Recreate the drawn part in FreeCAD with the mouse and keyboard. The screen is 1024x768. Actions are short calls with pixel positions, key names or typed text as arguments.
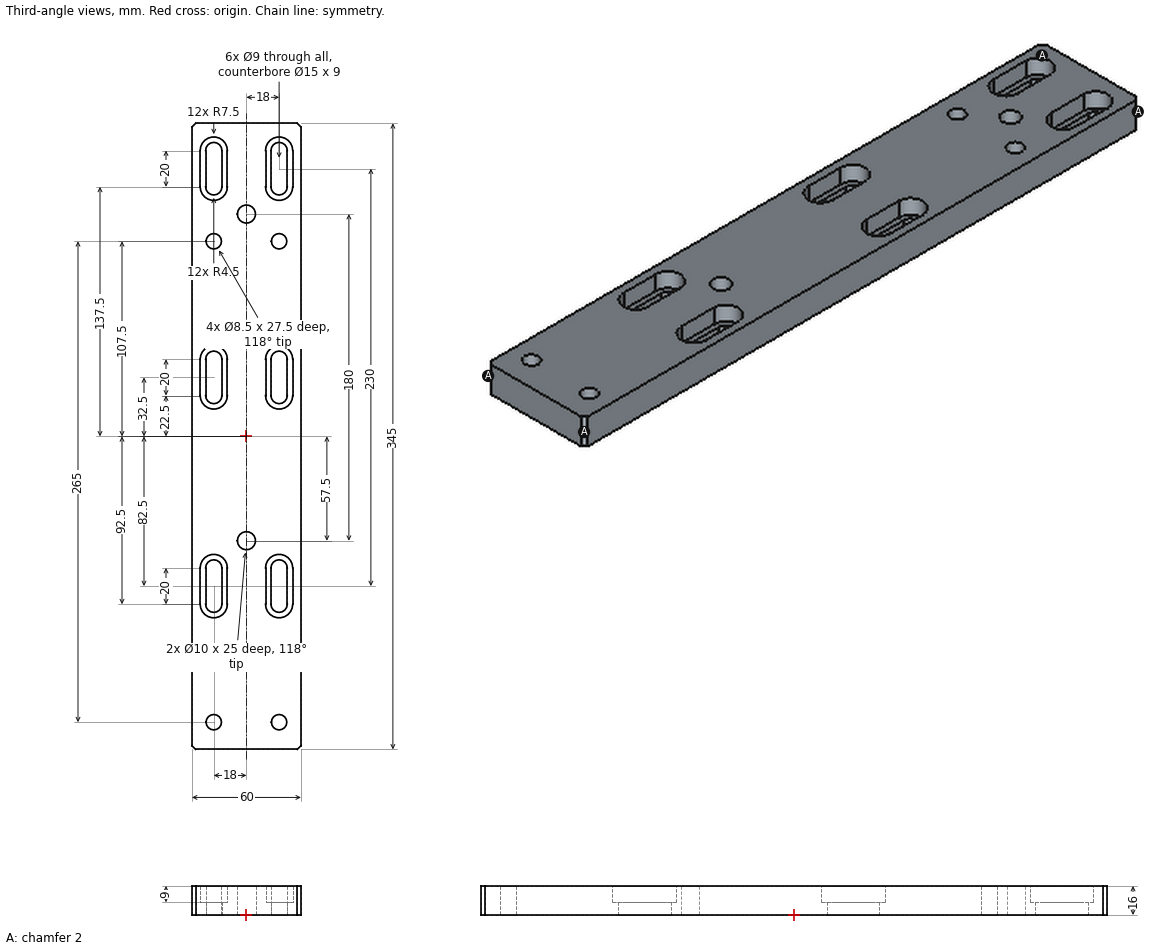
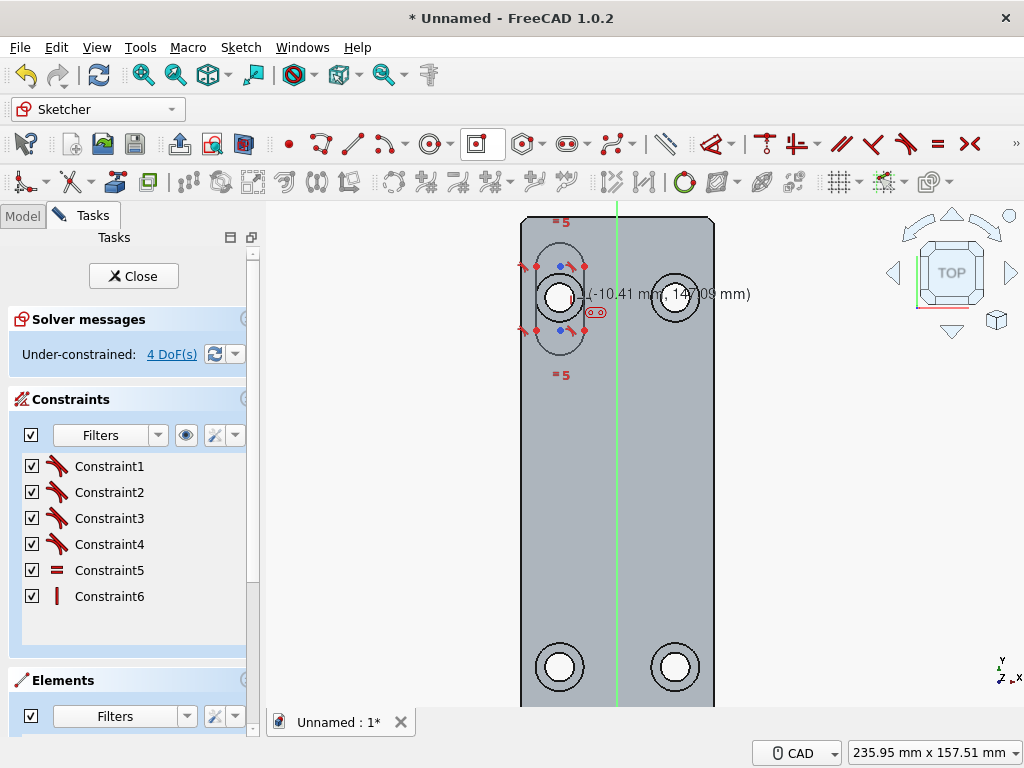
click(675, 330)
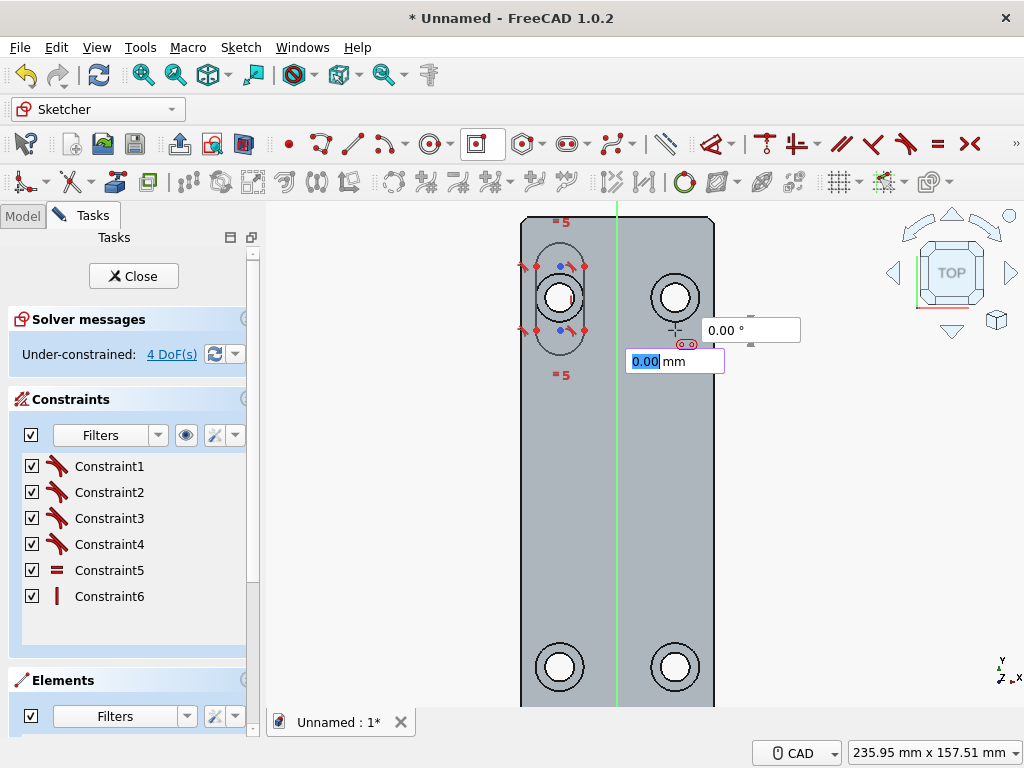
click(675, 266)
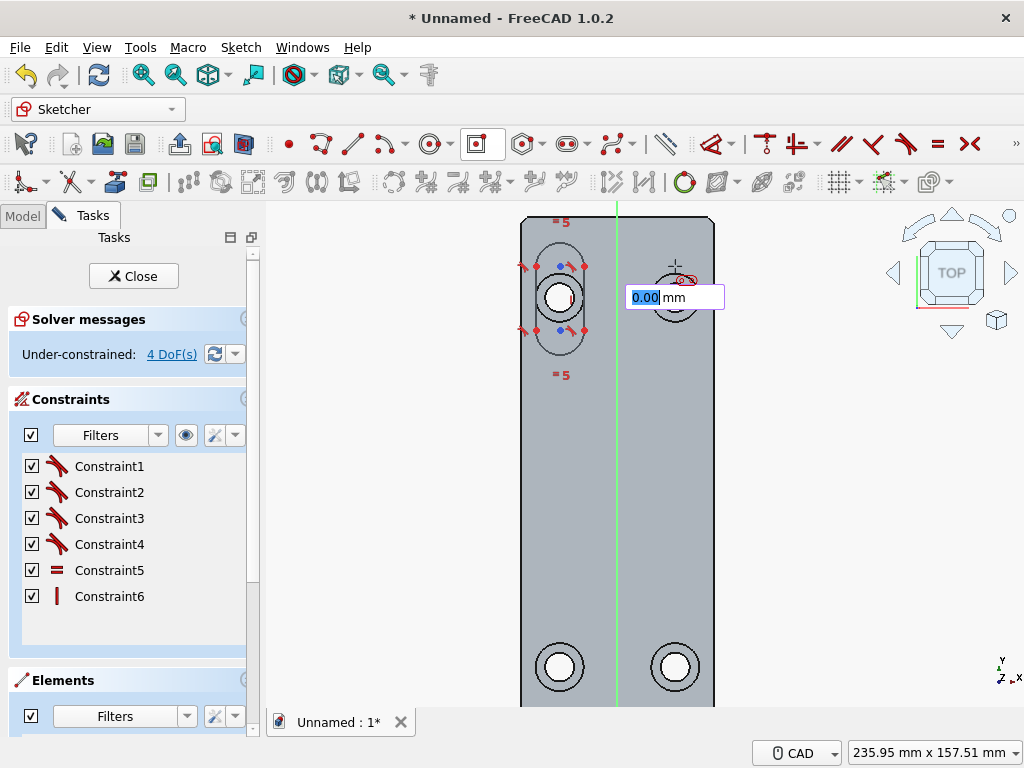
click(699, 298)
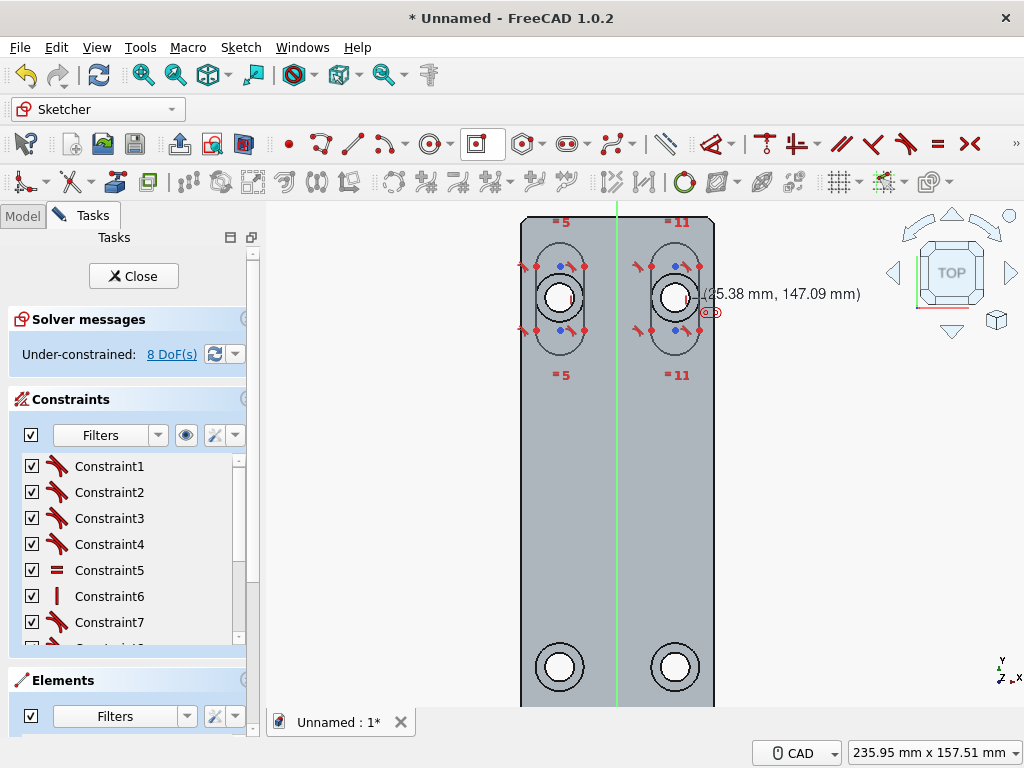
scroll(553, 330, down, 5)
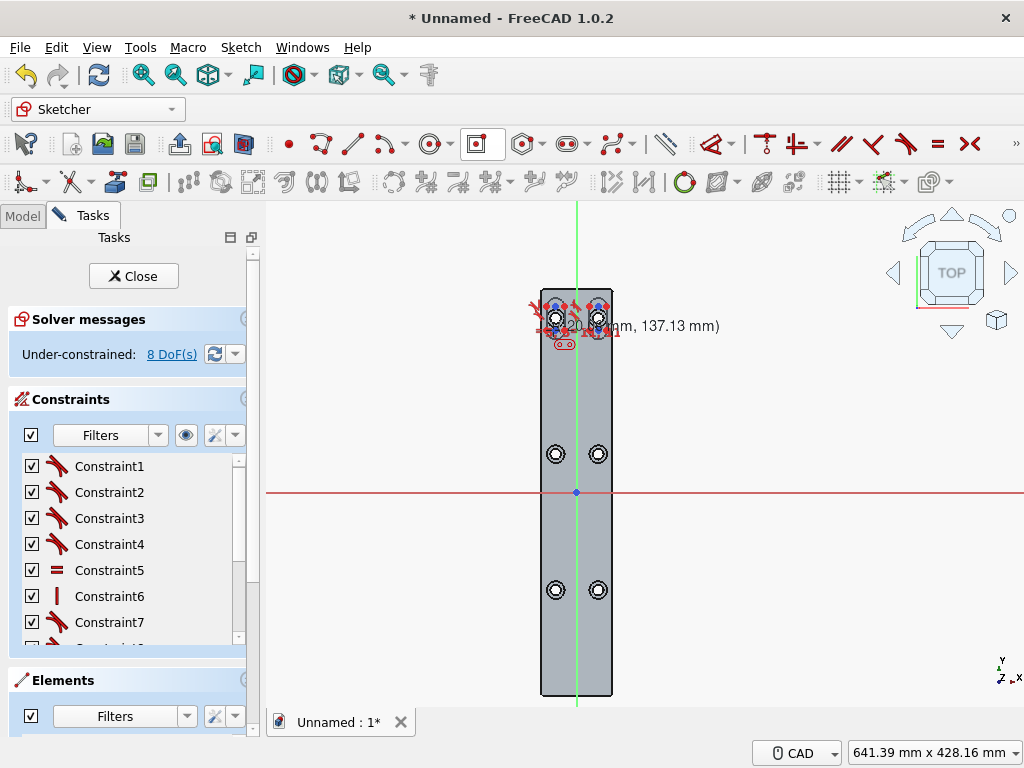
scroll(556, 466, up, 5)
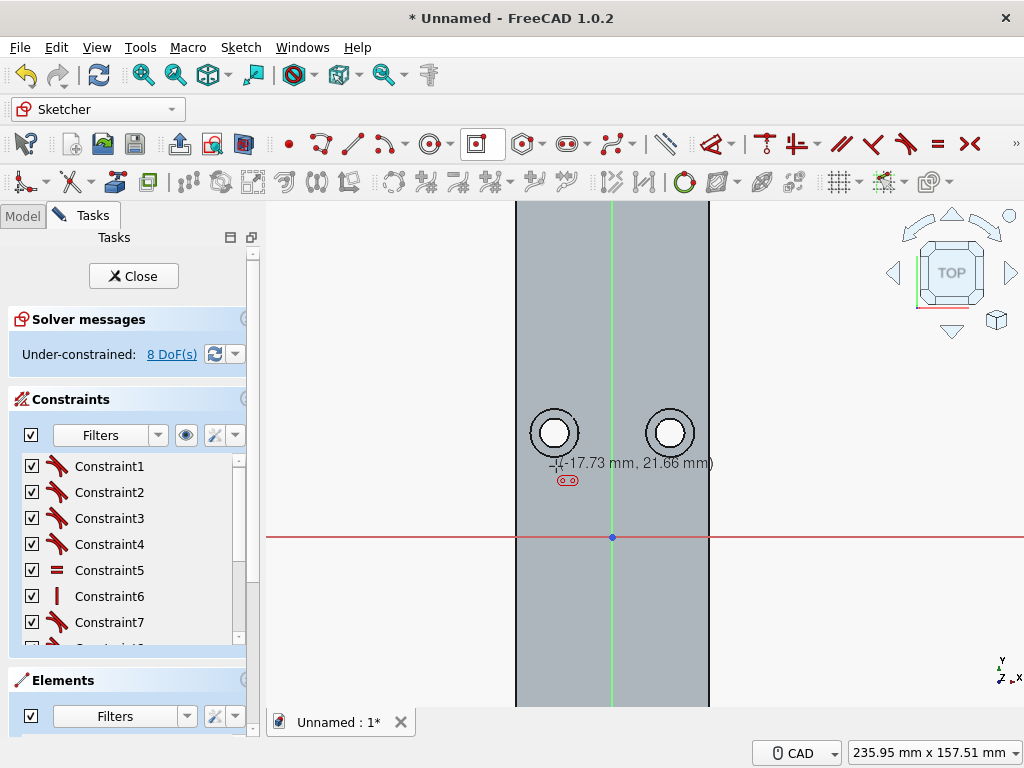
click(554, 465)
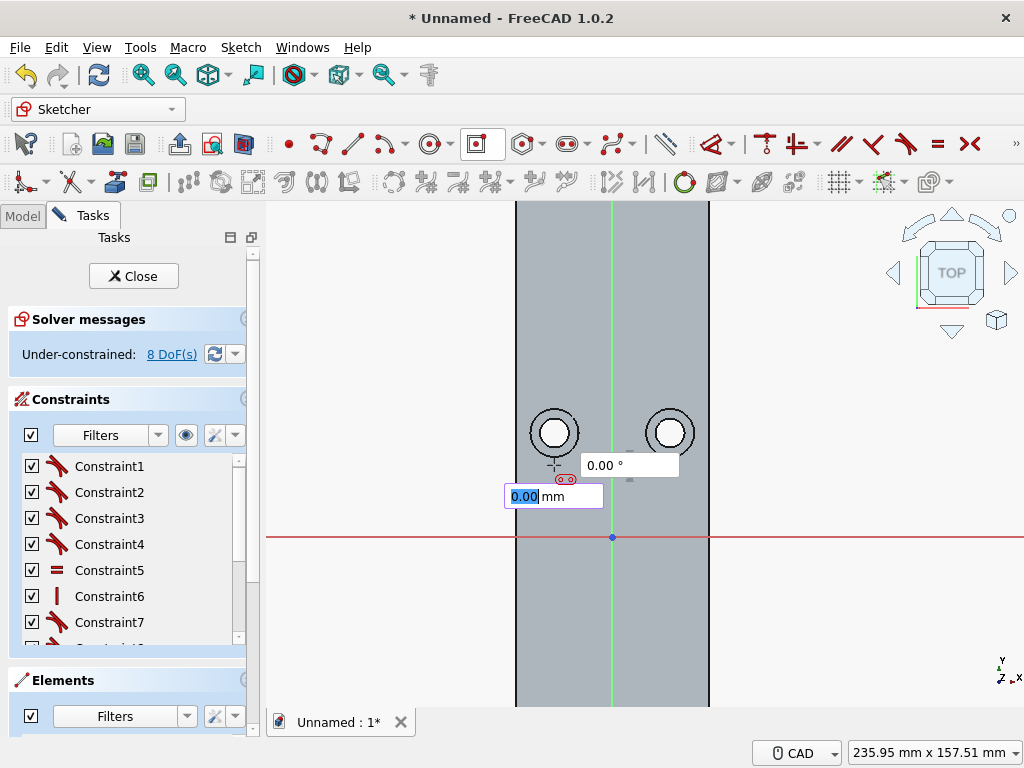
click(554, 401)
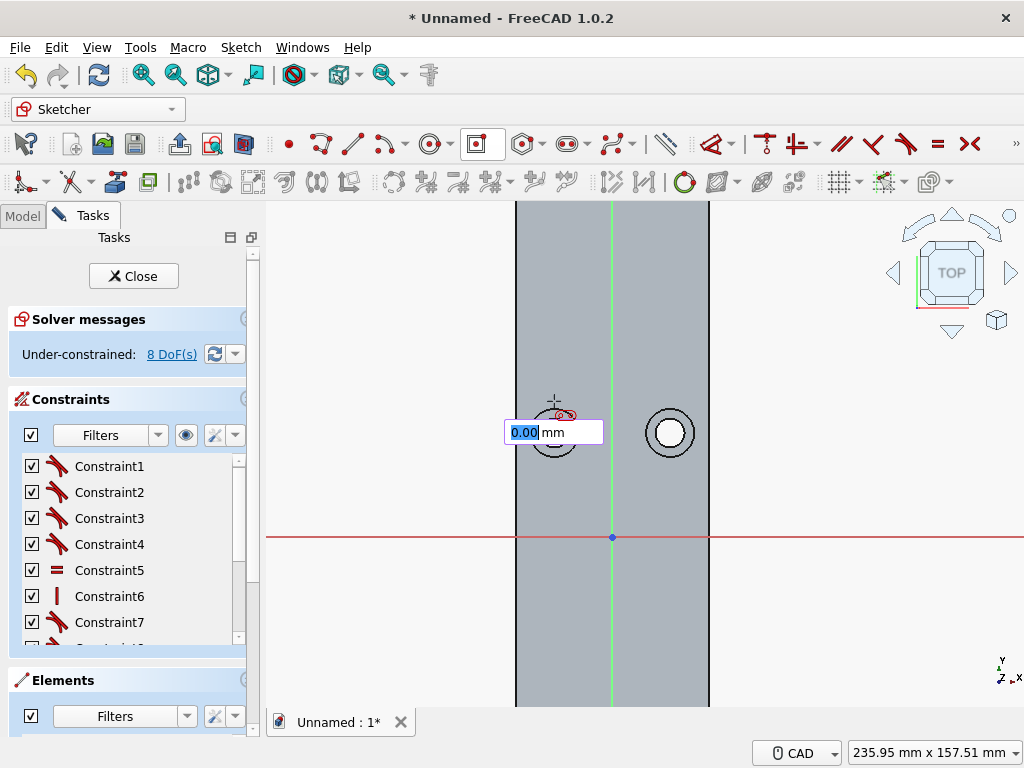
click(530, 433)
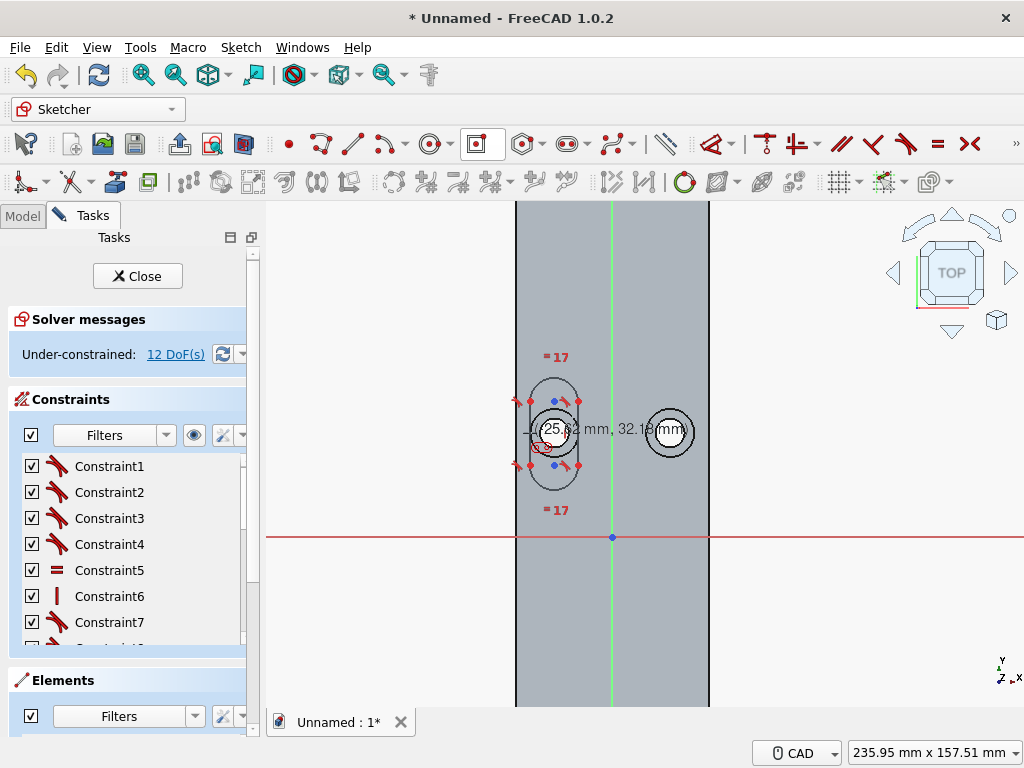
click(670, 465)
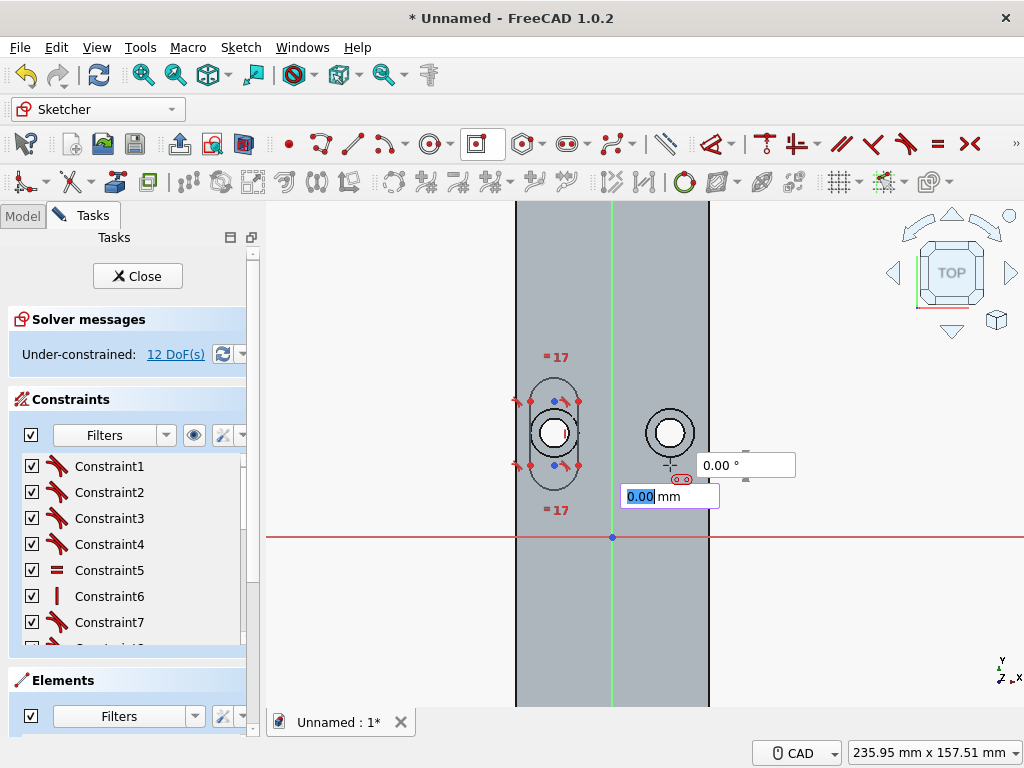
click(670, 401)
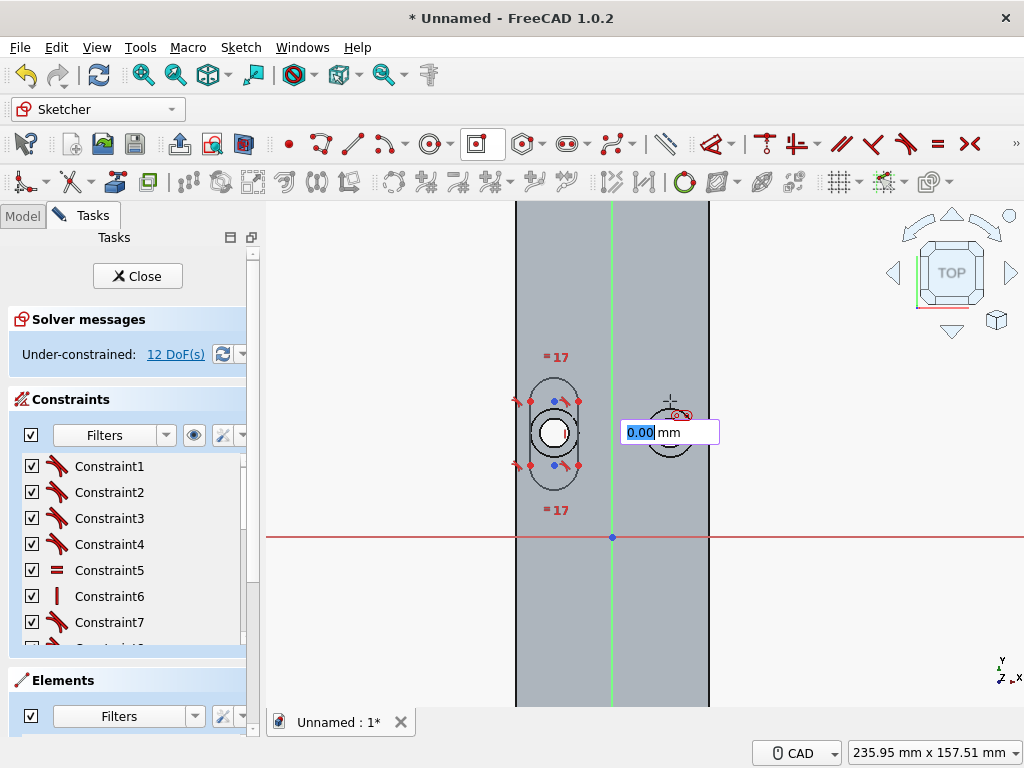
click(646, 433)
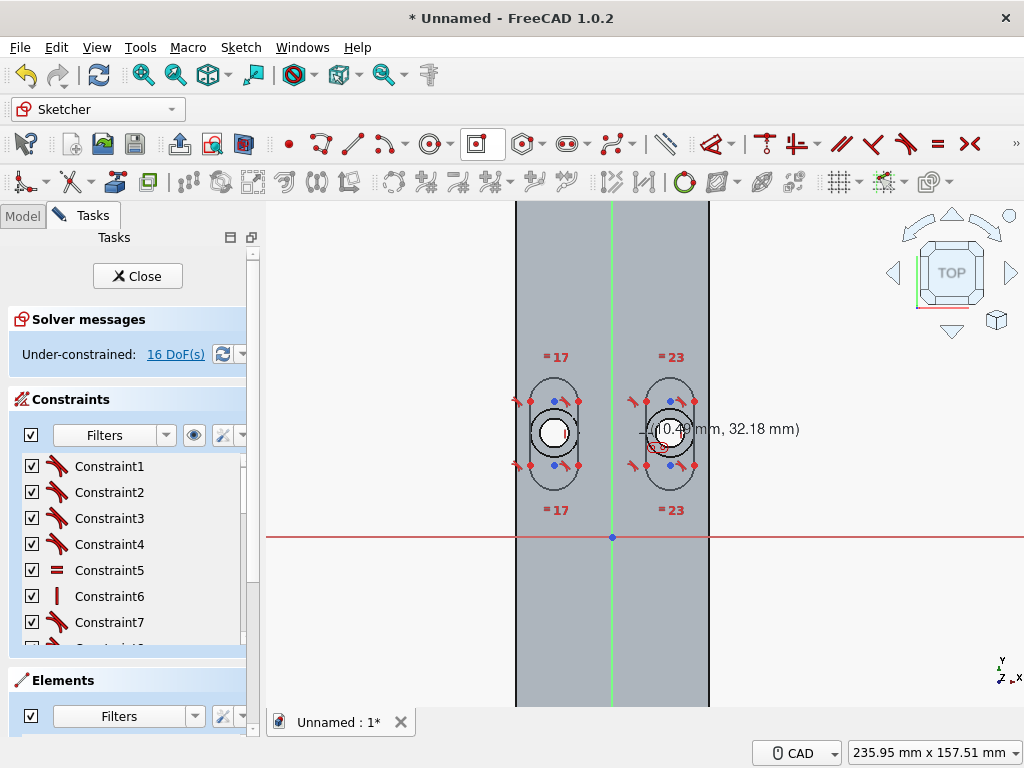
scroll(556, 466, down, 5)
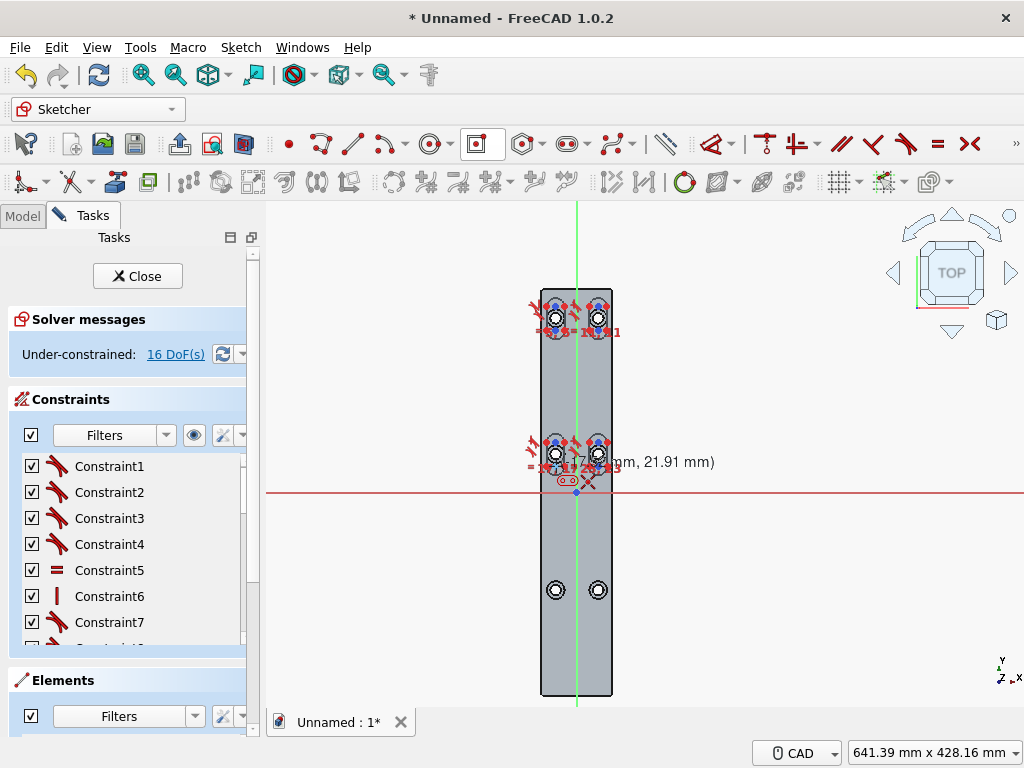
scroll(556, 602, up, 5)